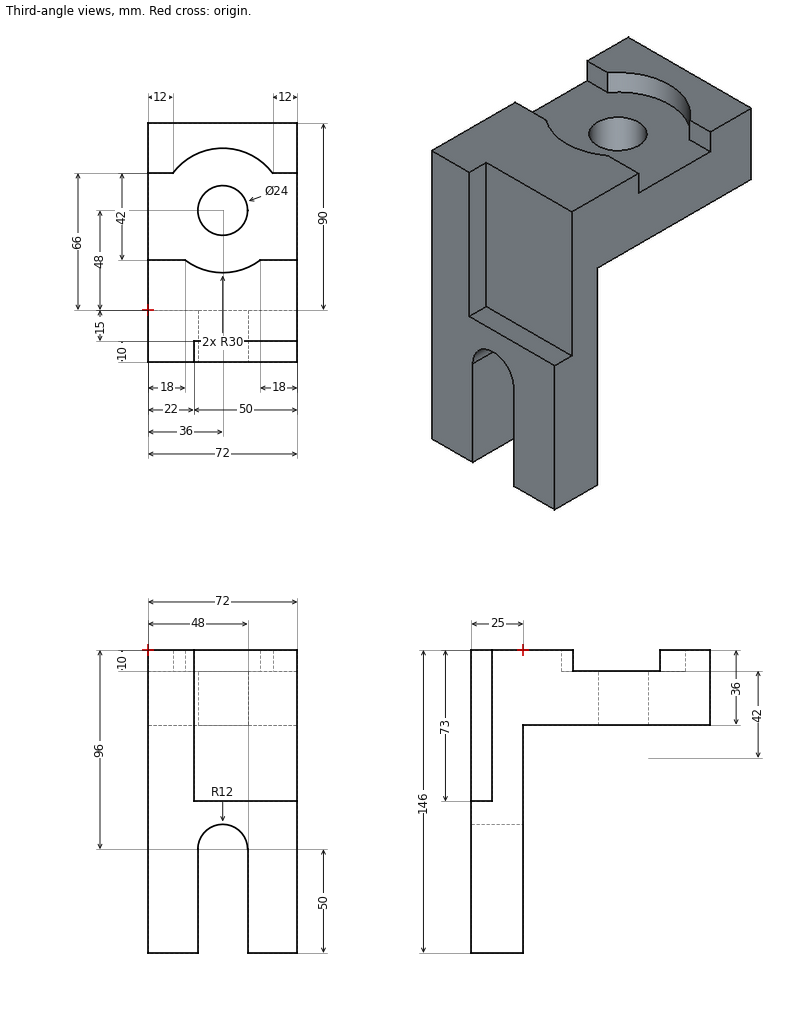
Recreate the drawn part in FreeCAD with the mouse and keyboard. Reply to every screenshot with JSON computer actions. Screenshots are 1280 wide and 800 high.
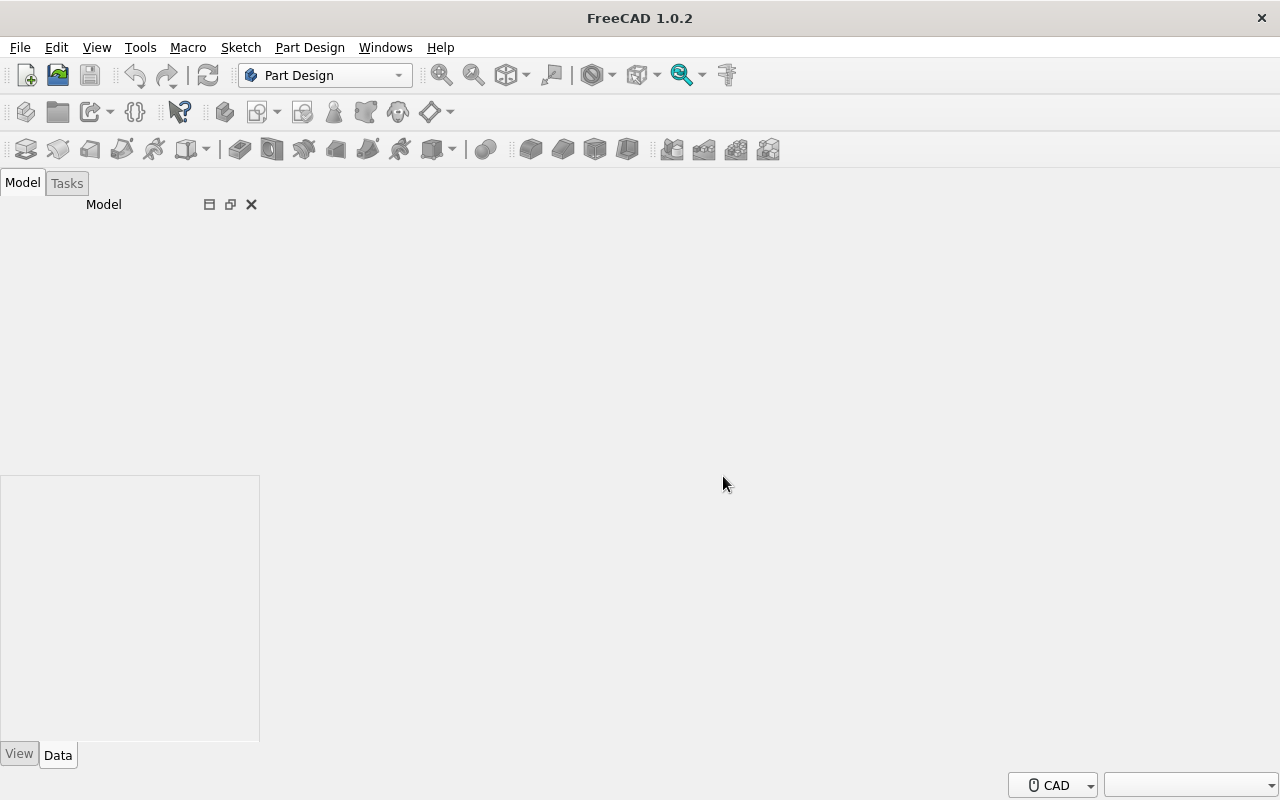
{"action": "key", "text": "ctrl+n"}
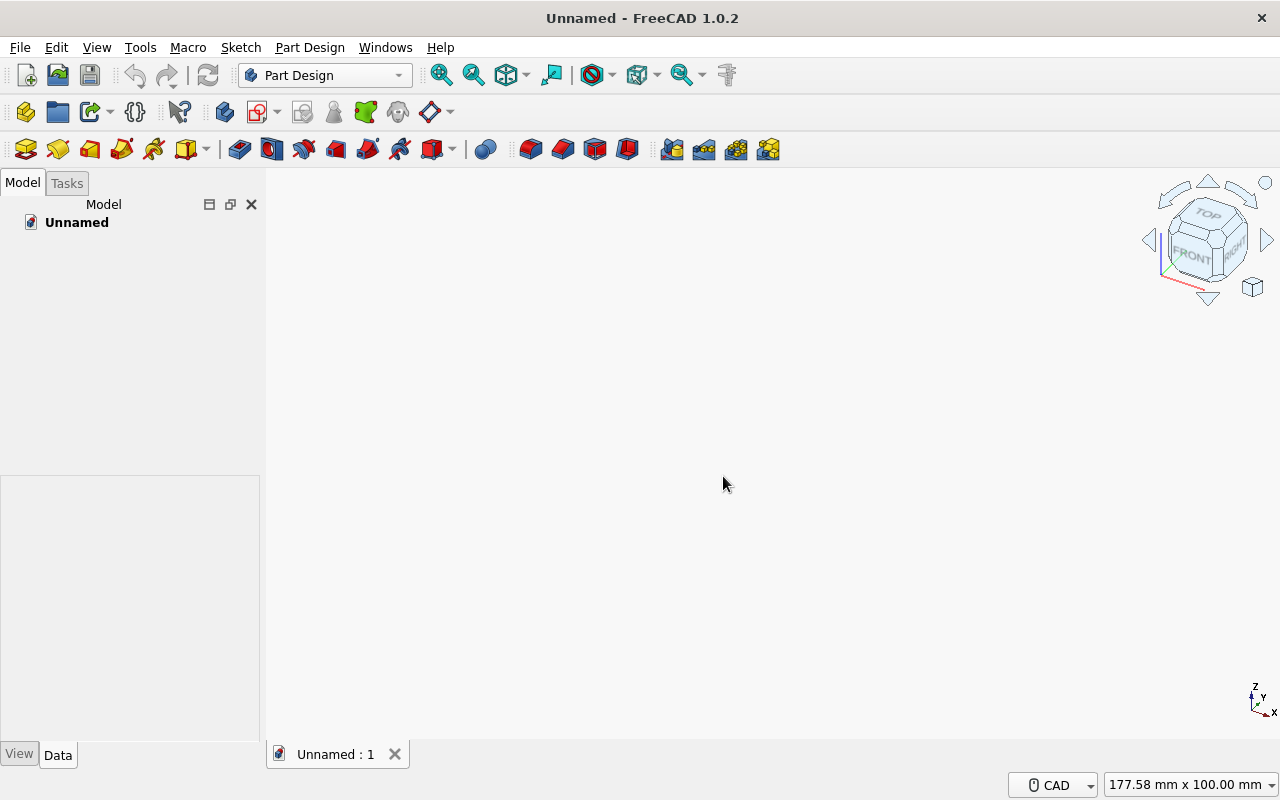
{"action": "left_click", "coordinate": [258, 112]}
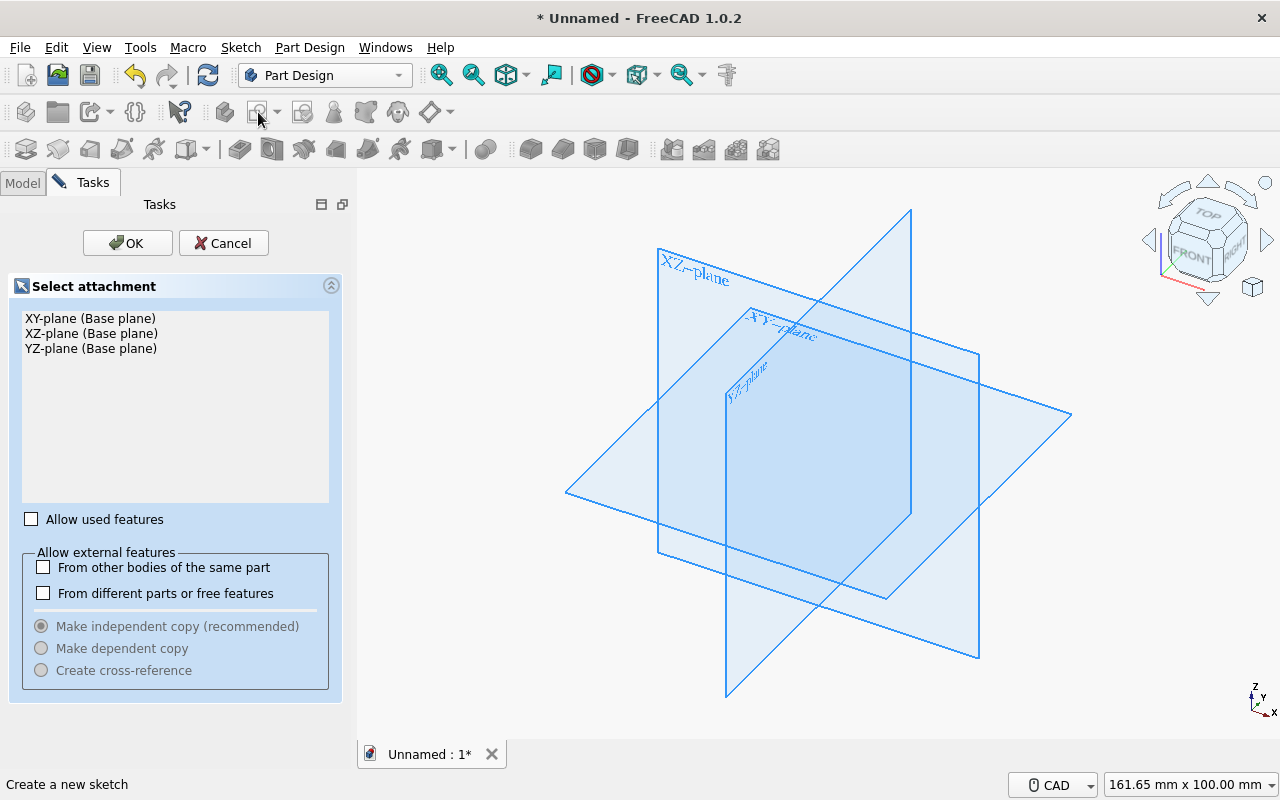
{"action": "left_click", "coordinate": [82, 318]}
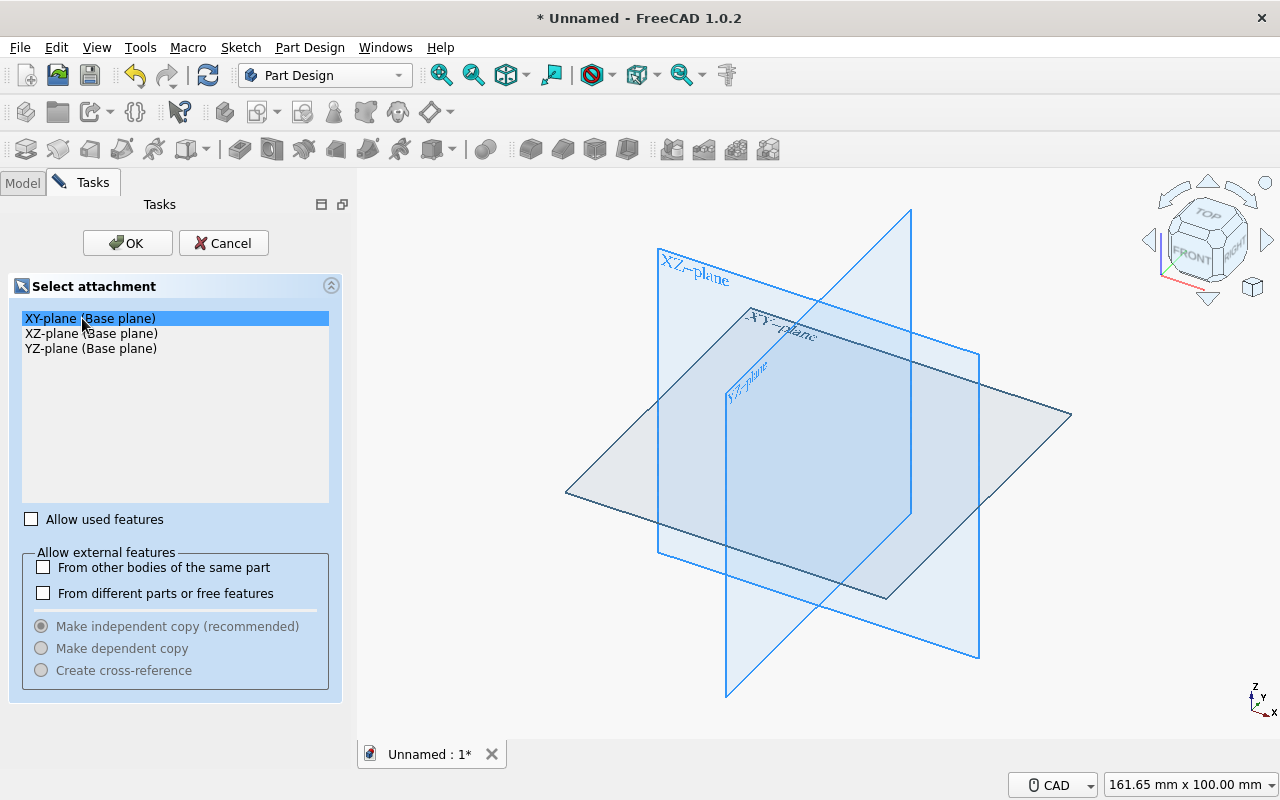
{"action": "left_click", "coordinate": [128, 243]}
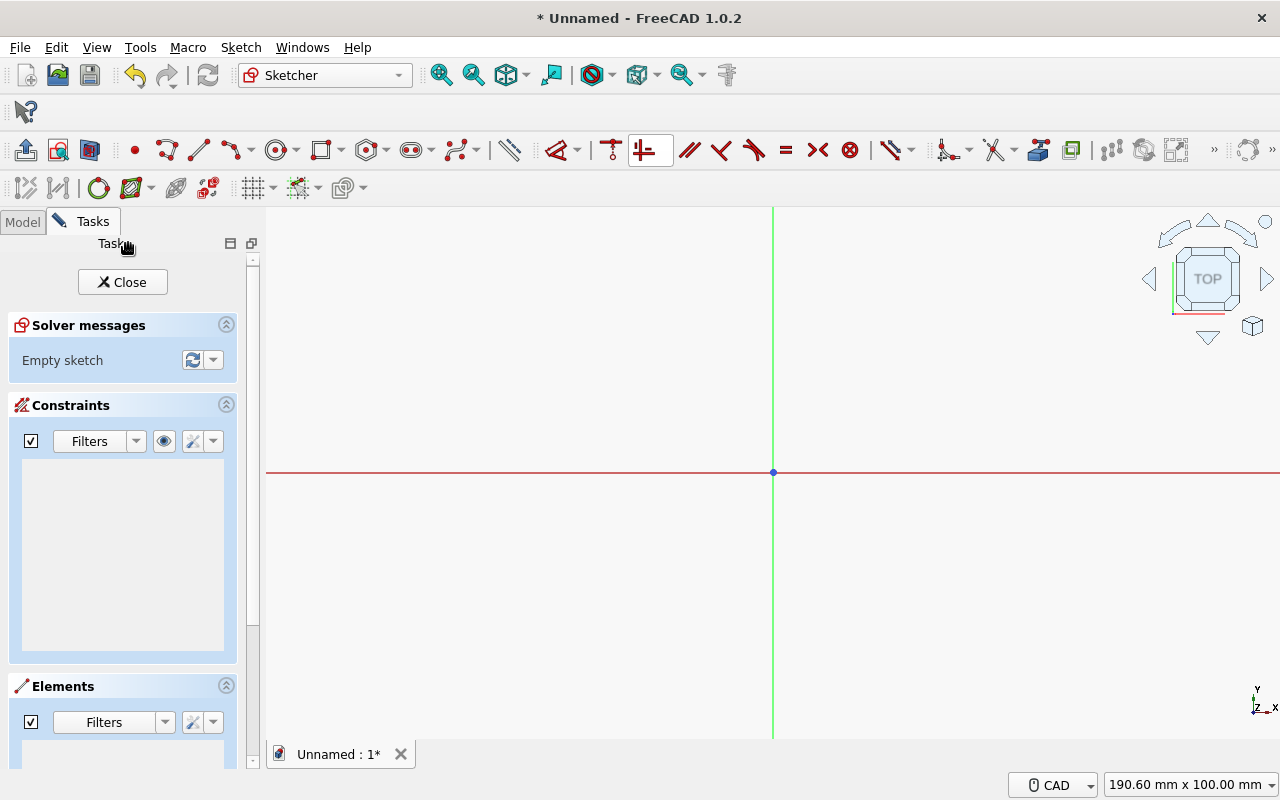
{"action": "scroll", "coordinate": [388, 711], "scroll_direction": "down", "scroll_amount": 3}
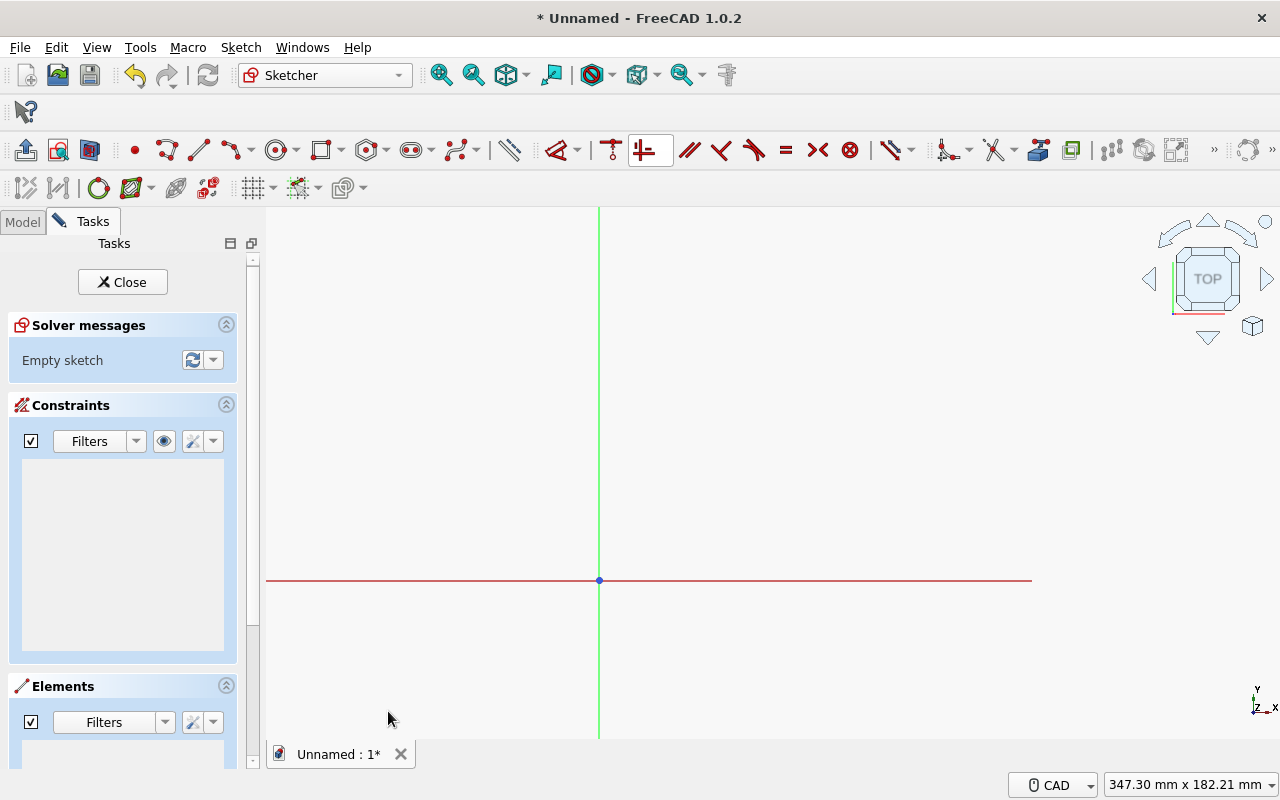
{"action": "left_click", "coordinate": [322, 150]}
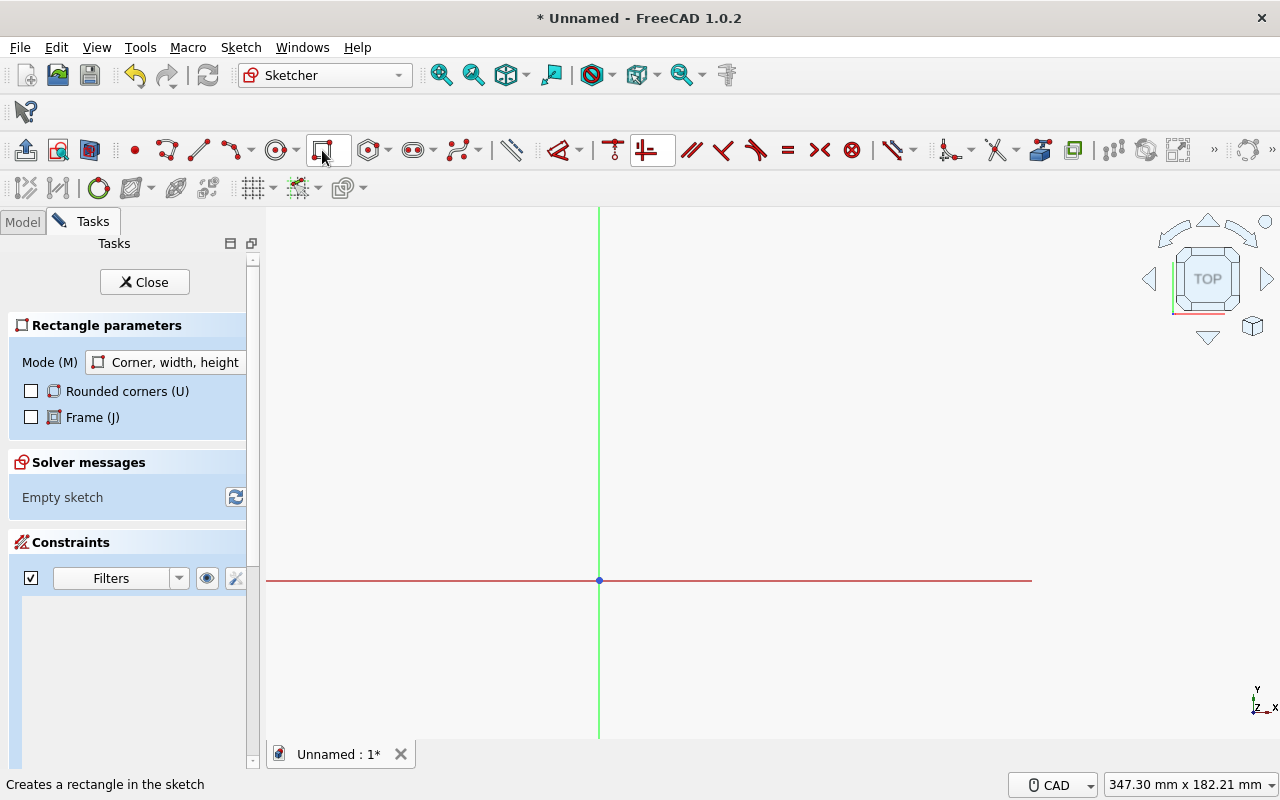
{"action": "left_click", "coordinate": [599, 581]}
{"action": "left_click", "coordinate": [810, 318]}
{"action": "key", "text": "Escape"}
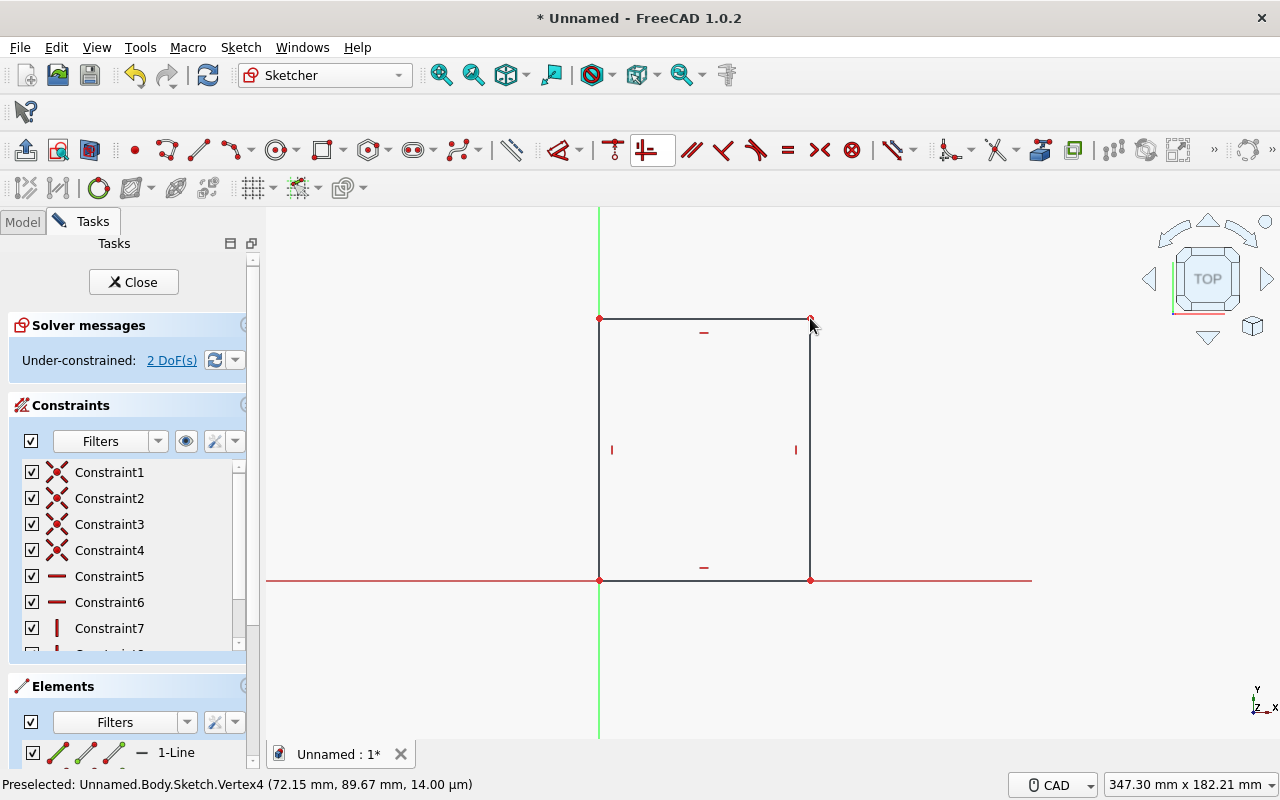
{"action": "left_click", "coordinate": [558, 150]}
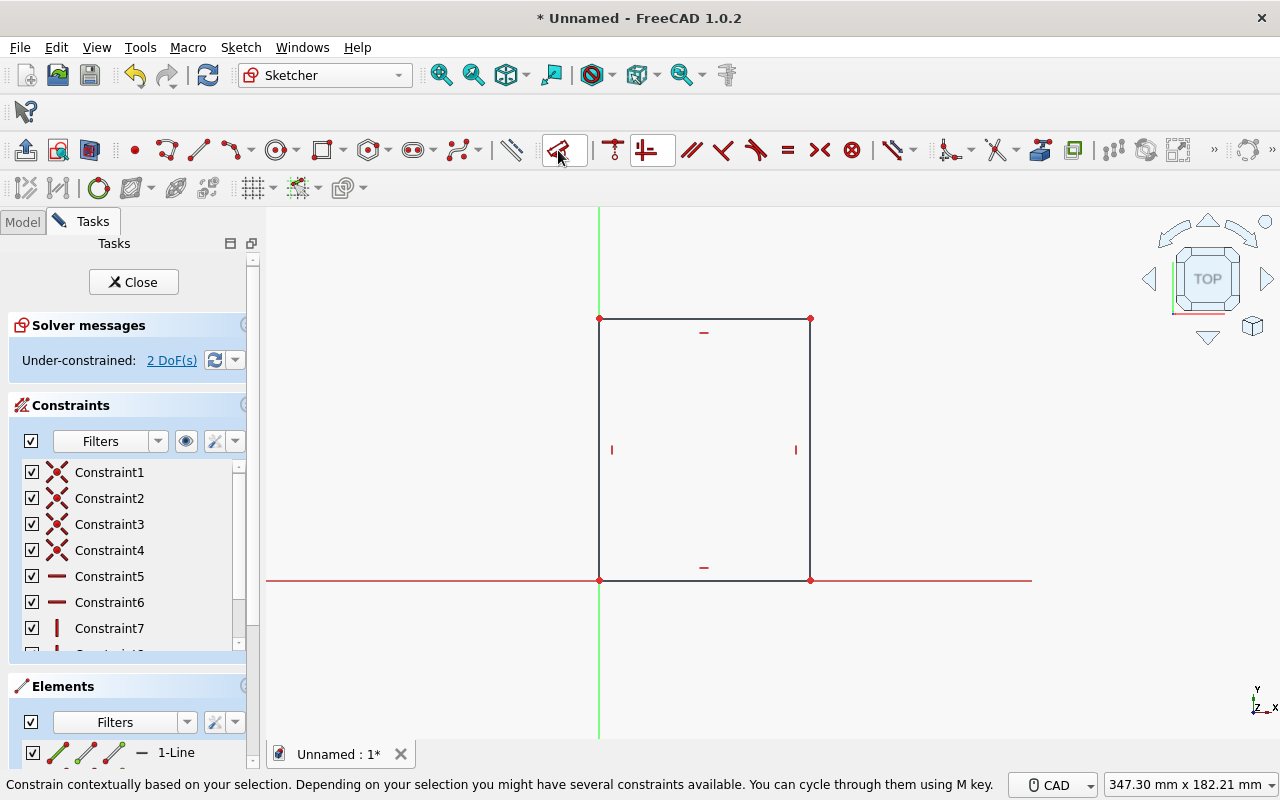
{"action": "left_click", "coordinate": [663, 581]}
{"action": "left_click", "coordinate": [705, 615]}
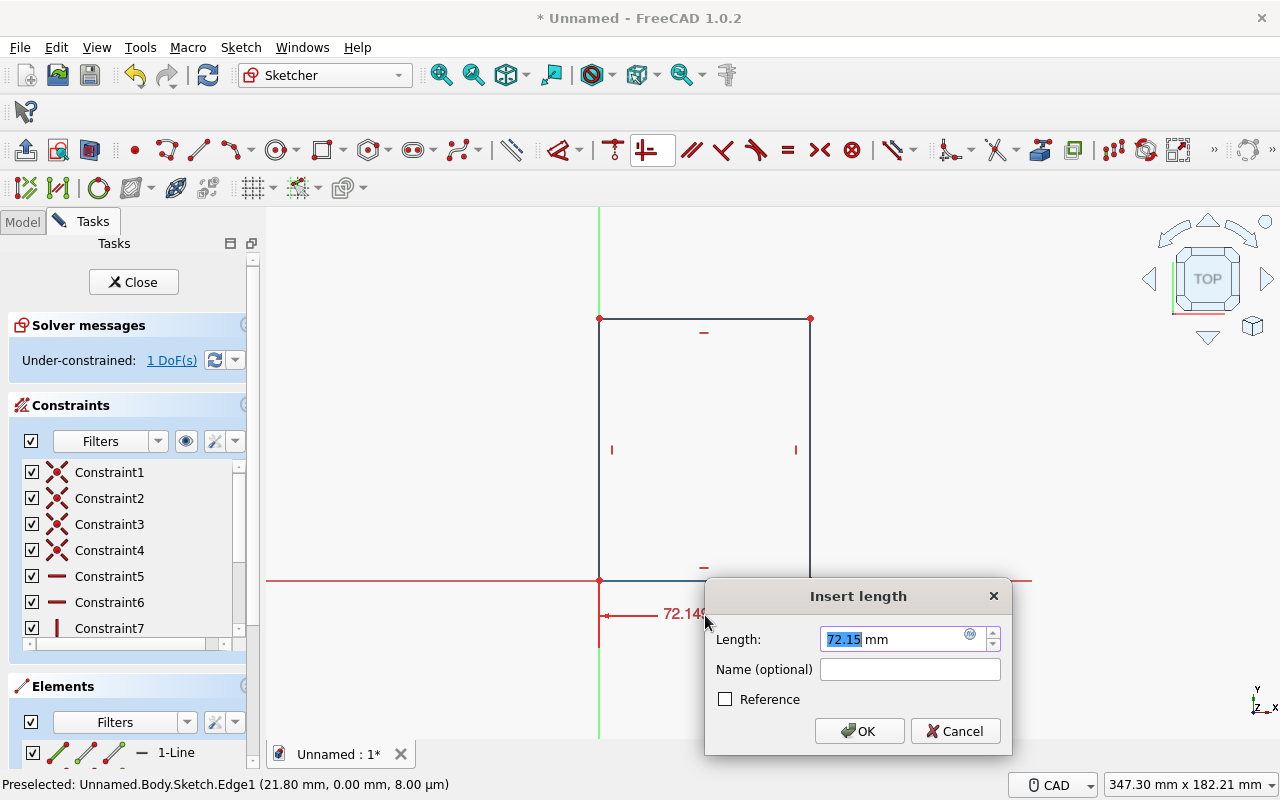
{"action": "type", "text": "72"}
{"action": "key", "text": "Return"}